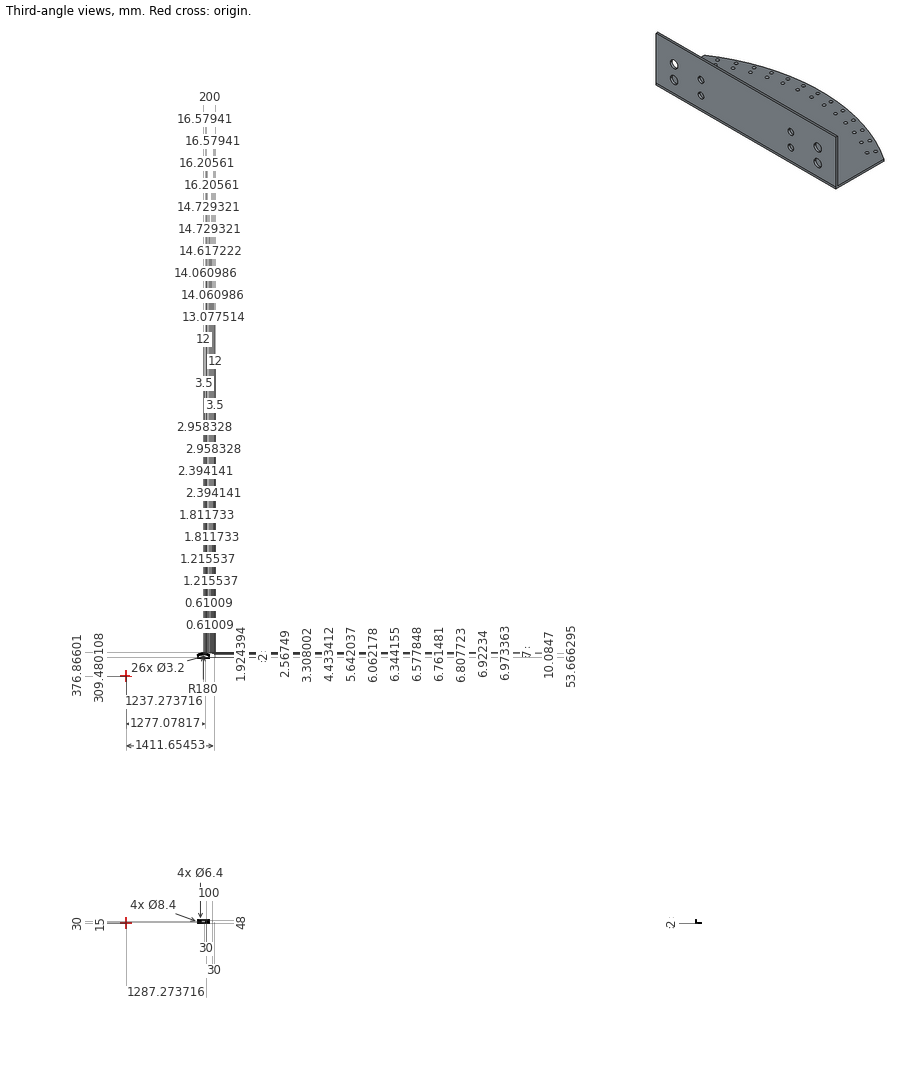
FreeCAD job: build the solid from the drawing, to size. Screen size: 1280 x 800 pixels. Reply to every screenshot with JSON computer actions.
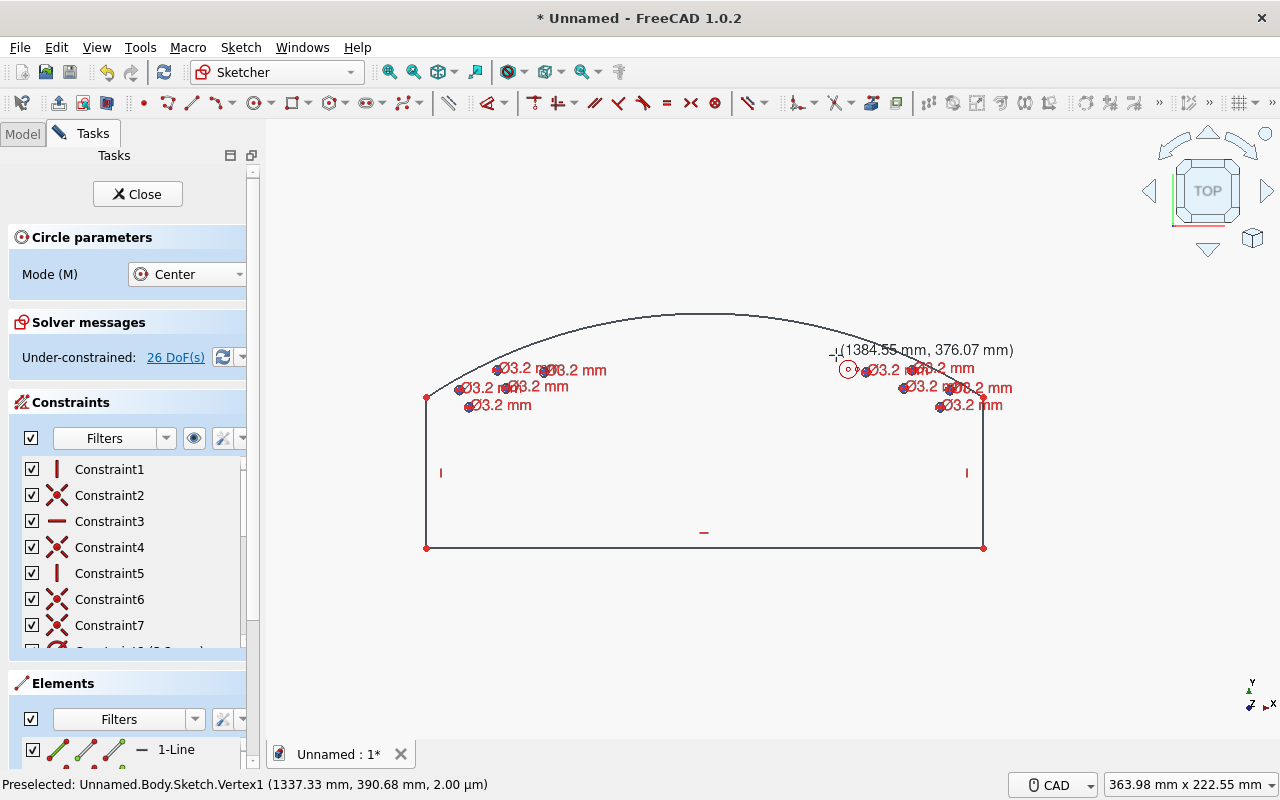
{"action": "scroll", "coordinate": [872, 353], "scroll_direction": "up", "scroll_amount": 2}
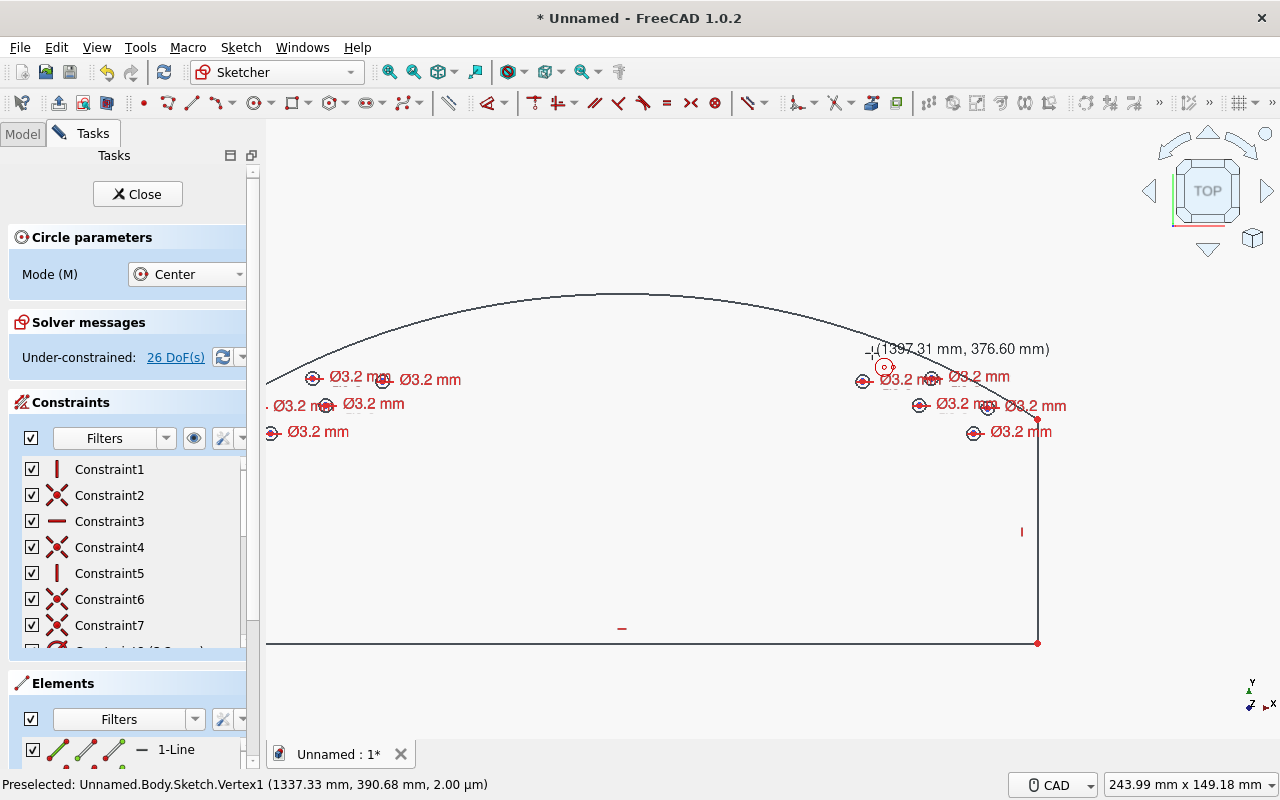
{"action": "left_click", "coordinate": [872, 353]}
{"action": "mouse_move", "coordinate": [877, 358]}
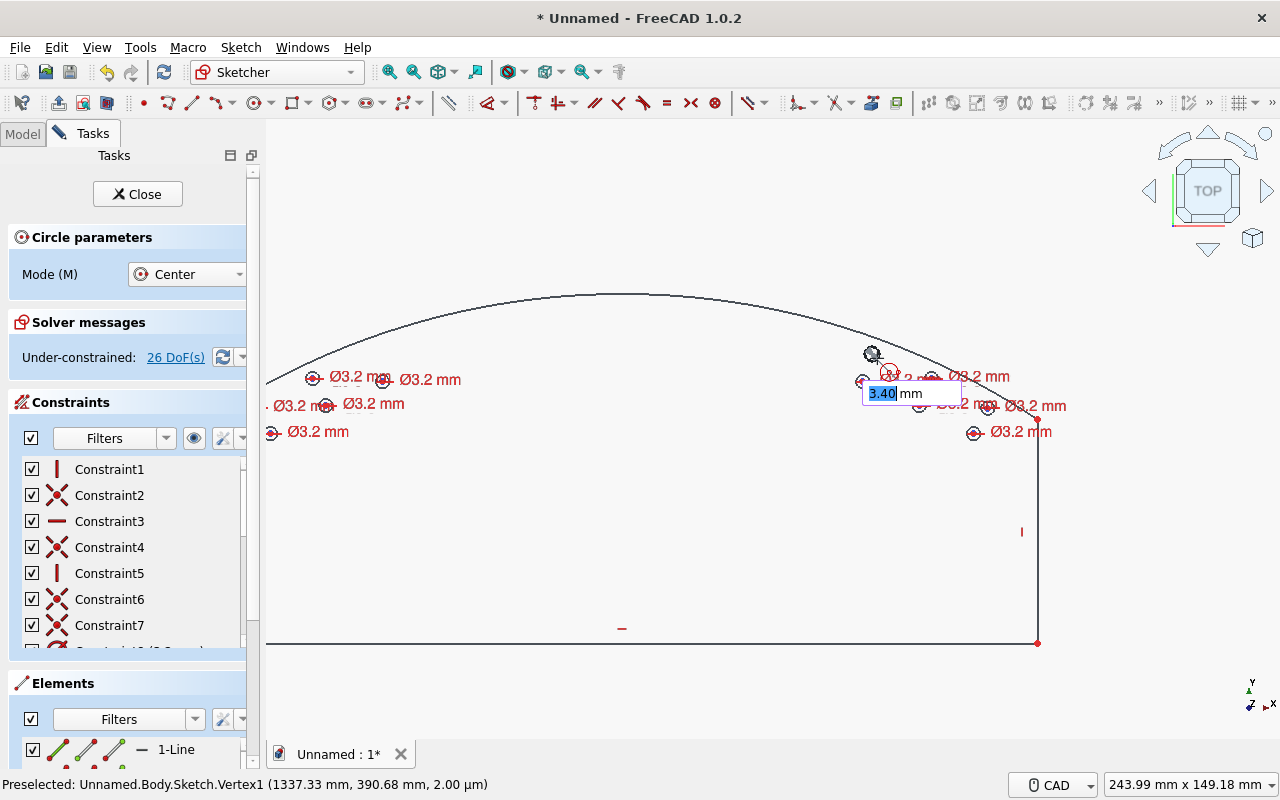
{"action": "type", "text": "3.2"}
{"action": "key", "text": "Return"}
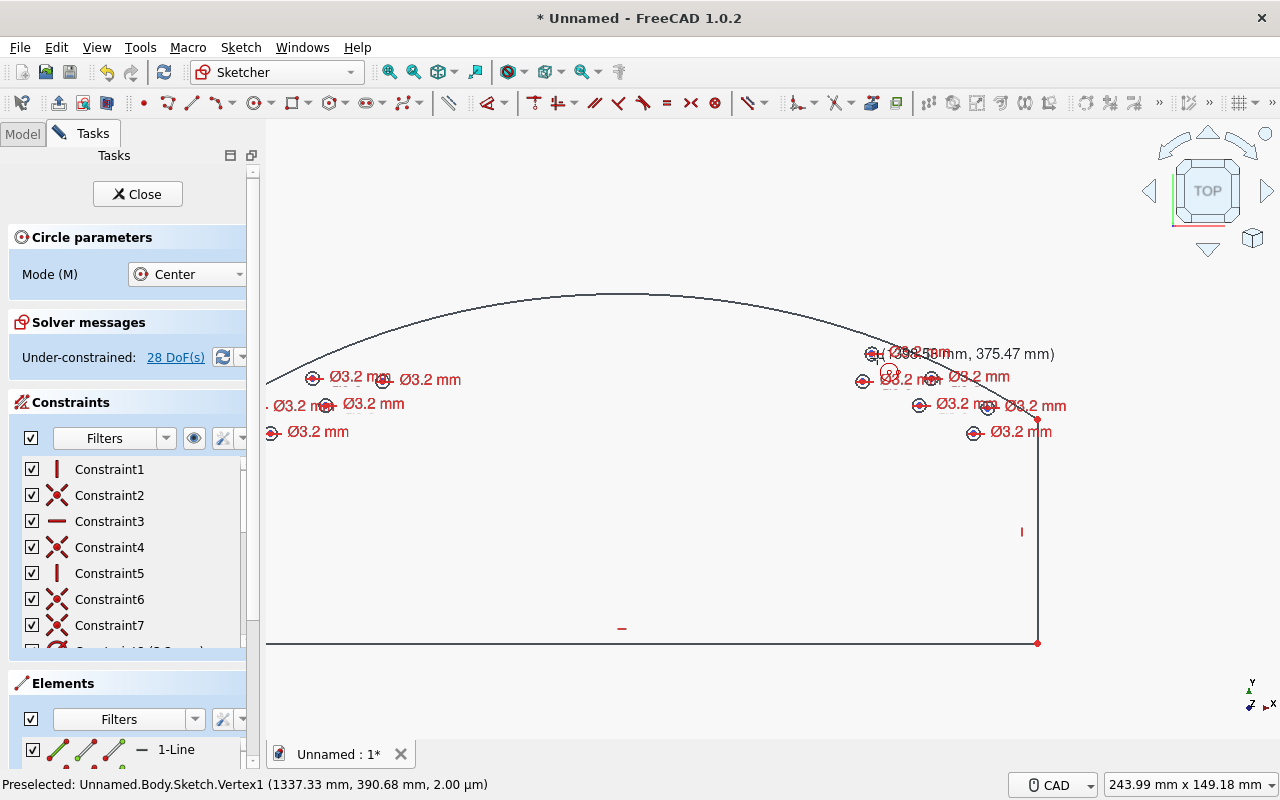
{"action": "scroll", "coordinate": [804, 362], "scroll_direction": "up", "scroll_amount": 7}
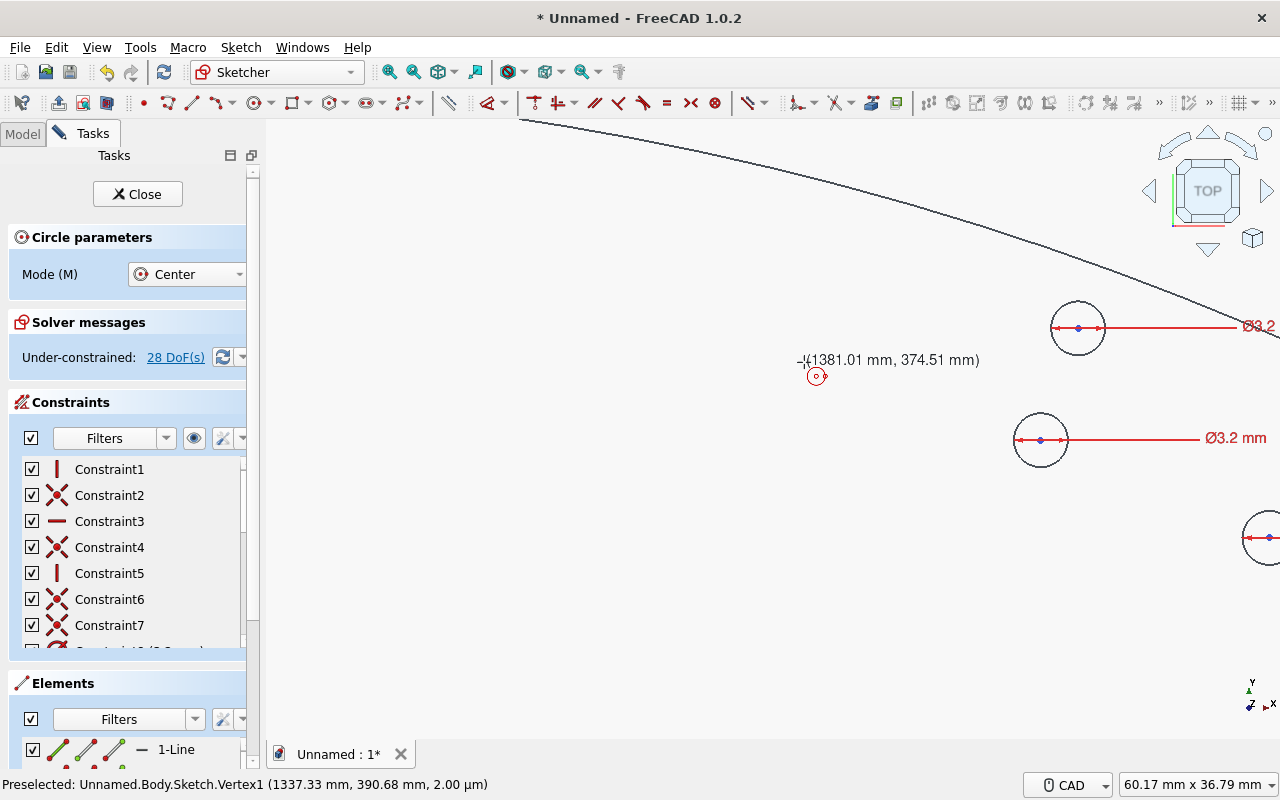
{"action": "scroll", "coordinate": [831, 358], "scroll_direction": "down", "scroll_amount": 9}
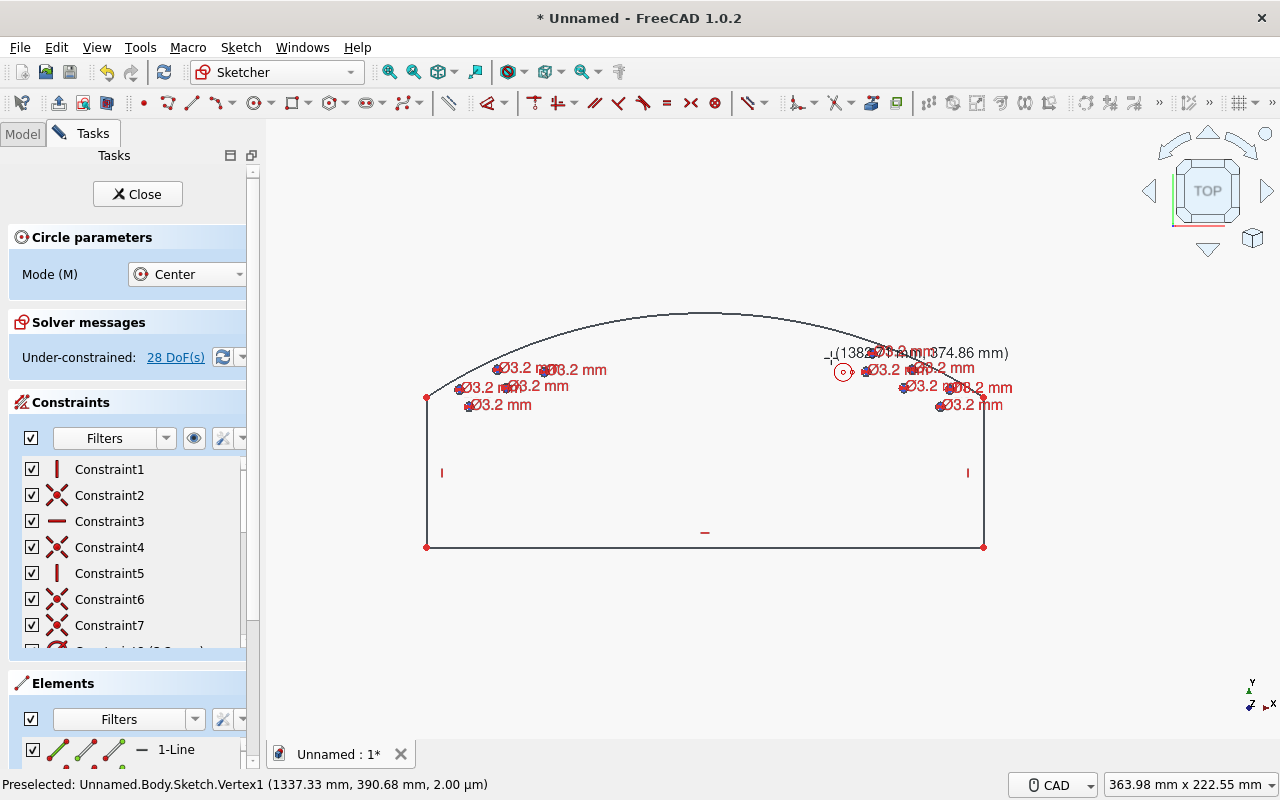
{"action": "left_click", "coordinate": [827, 359]}
{"action": "mouse_move", "coordinate": [830, 356]}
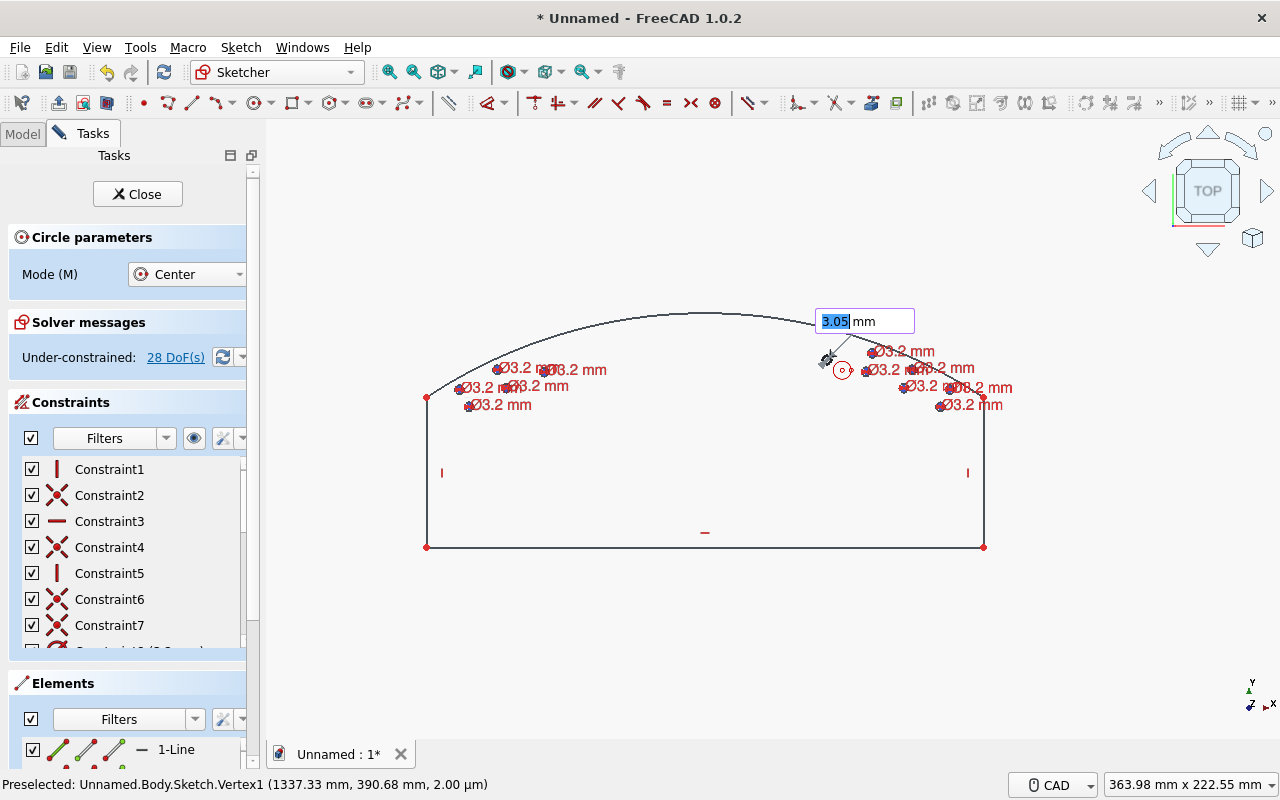
{"action": "type", "text": "3.2"}
{"action": "key", "text": "Return"}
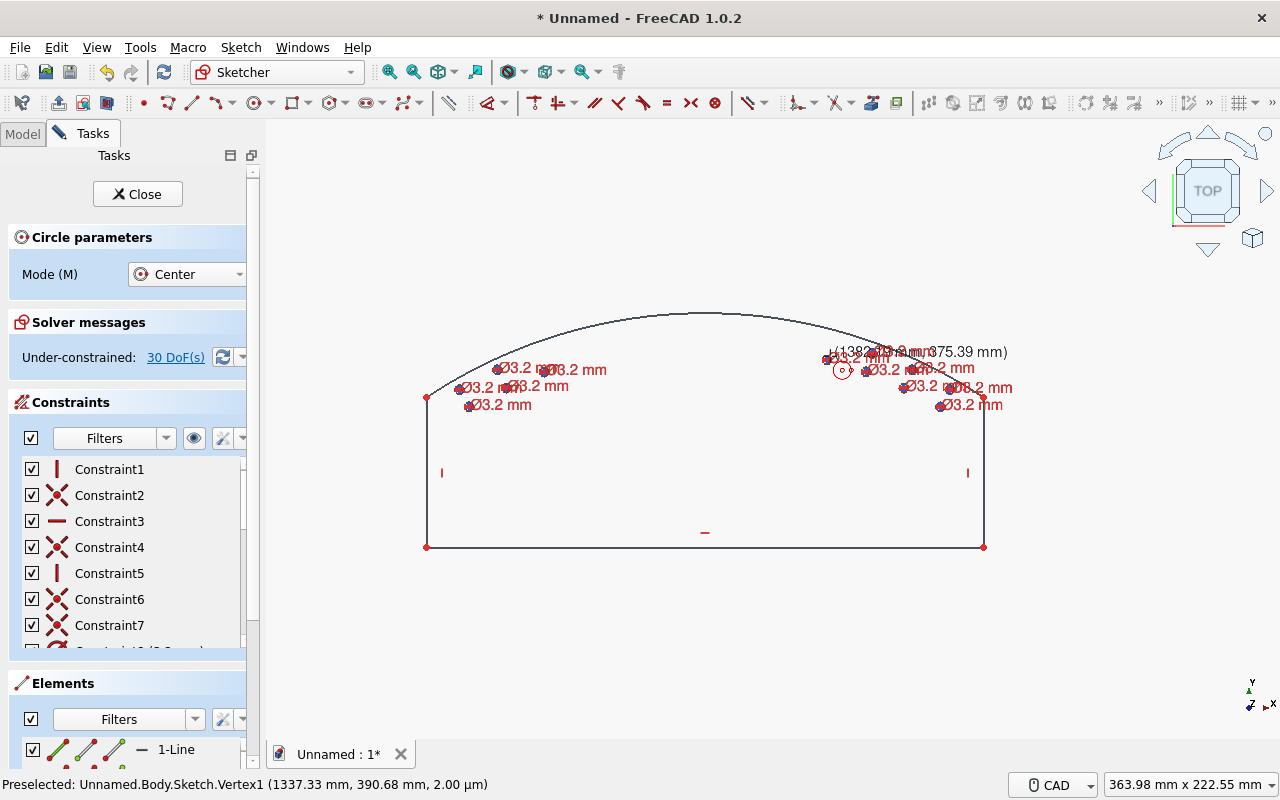
{"action": "scroll", "coordinate": [787, 350], "scroll_direction": "up", "scroll_amount": 9}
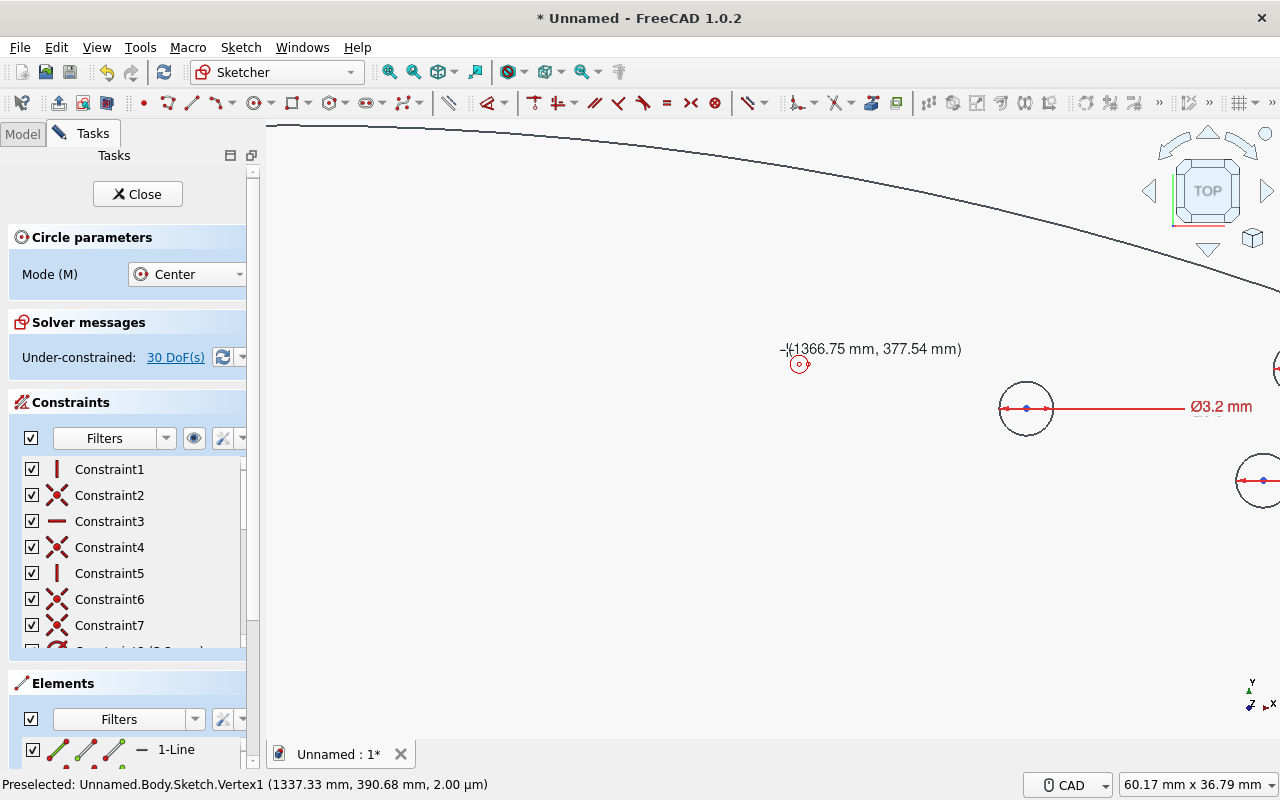
{"action": "scroll", "coordinate": [787, 350], "scroll_direction": "down", "scroll_amount": 9}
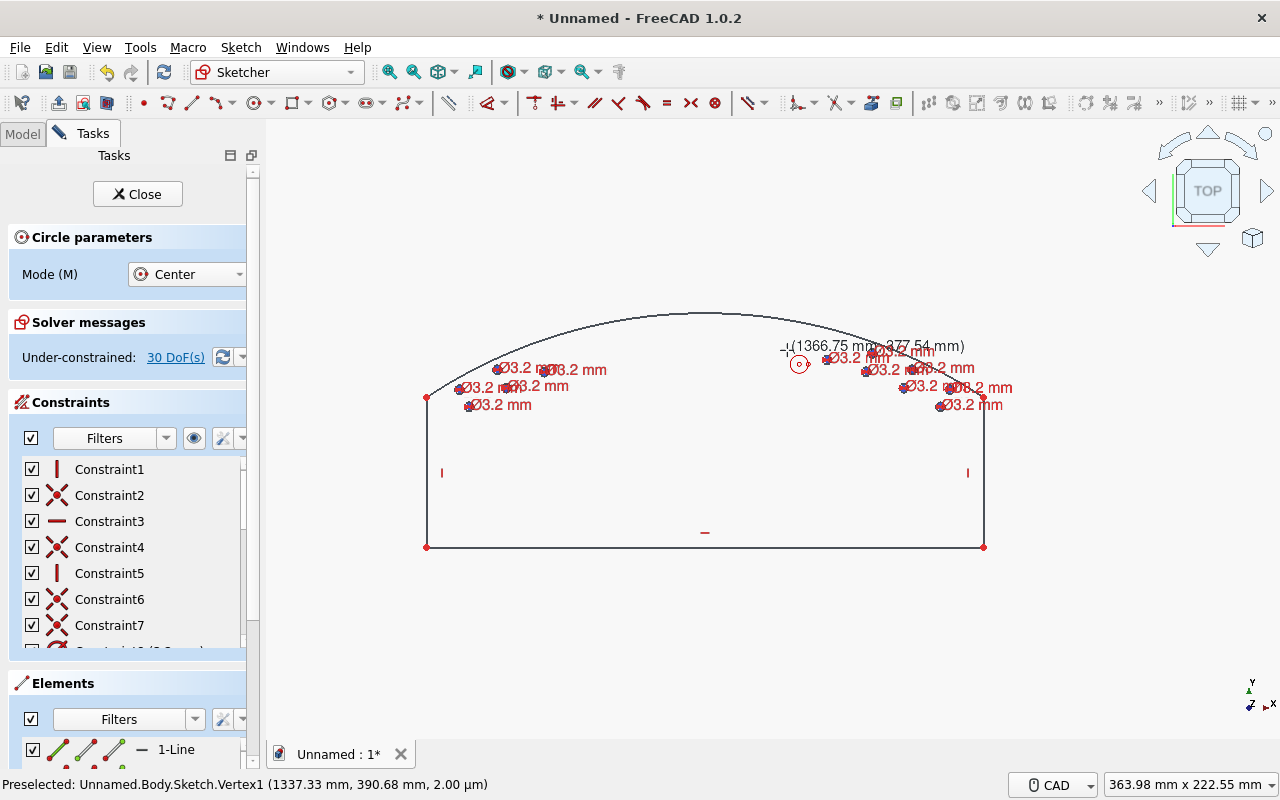
{"action": "left_click", "coordinate": [787, 350]}
{"action": "mouse_move", "coordinate": [790, 347]}